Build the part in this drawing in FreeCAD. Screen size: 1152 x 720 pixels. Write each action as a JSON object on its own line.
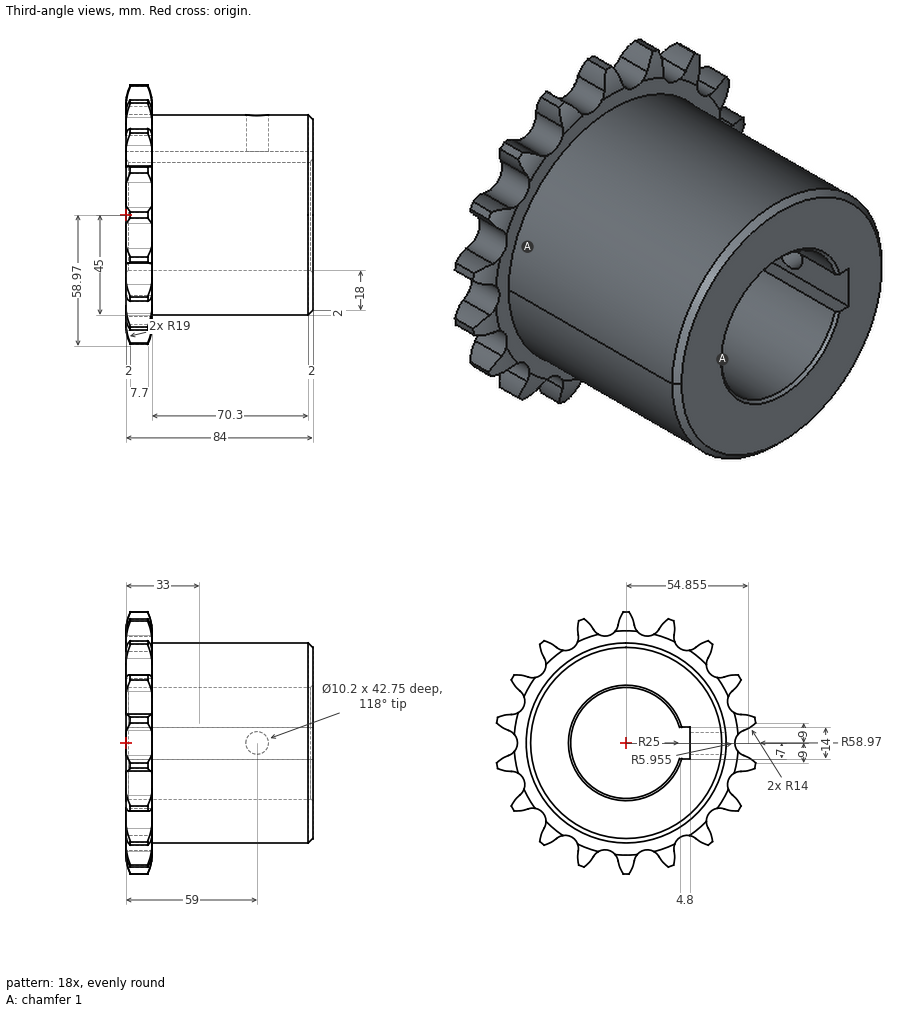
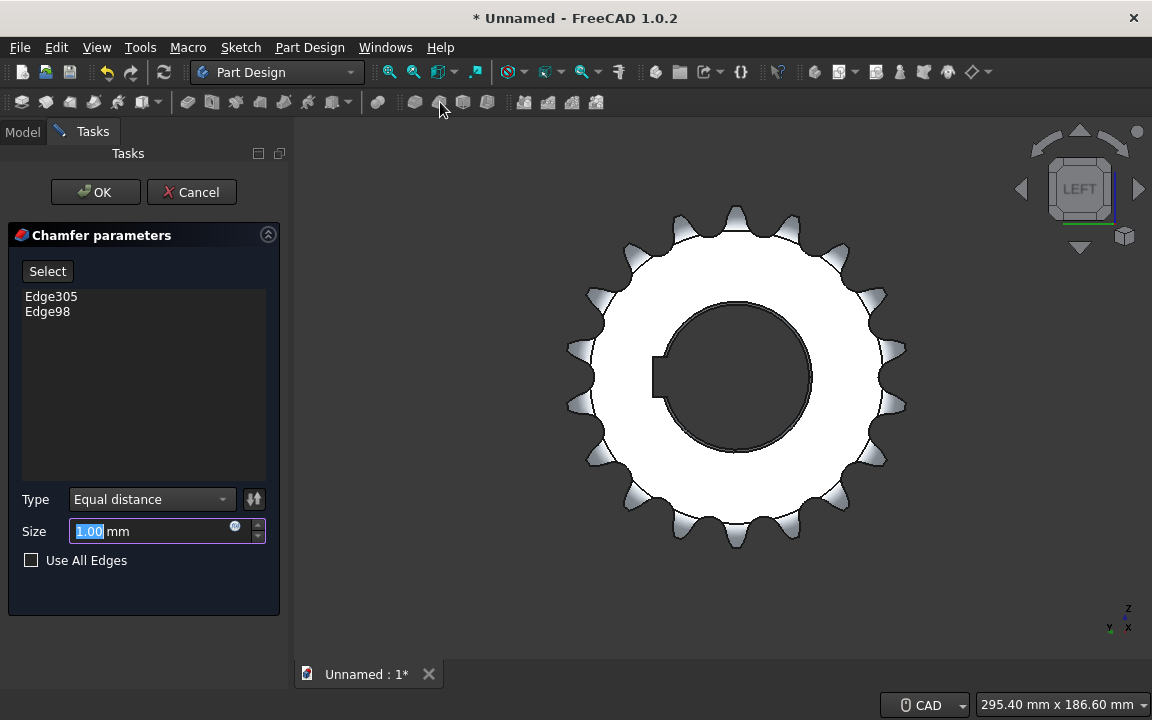
{"action": "type", "text": "1"}
{"action": "key", "text": "Tab"}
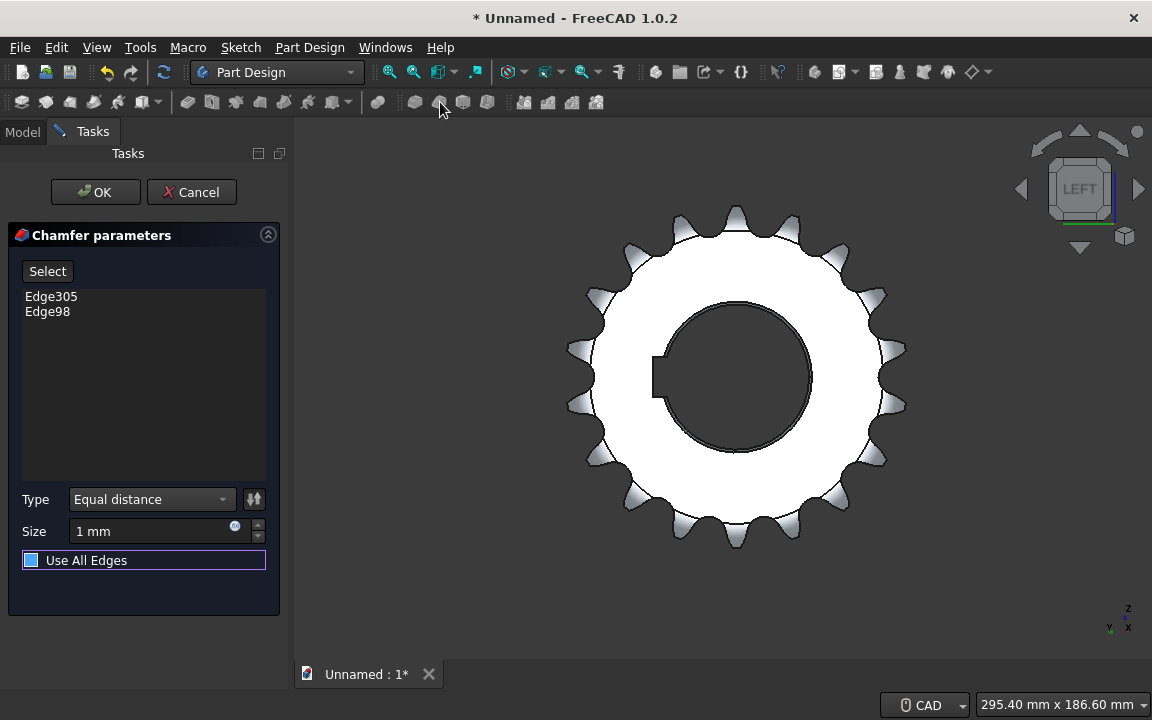
{"action": "left_click", "coordinate": [96, 192]}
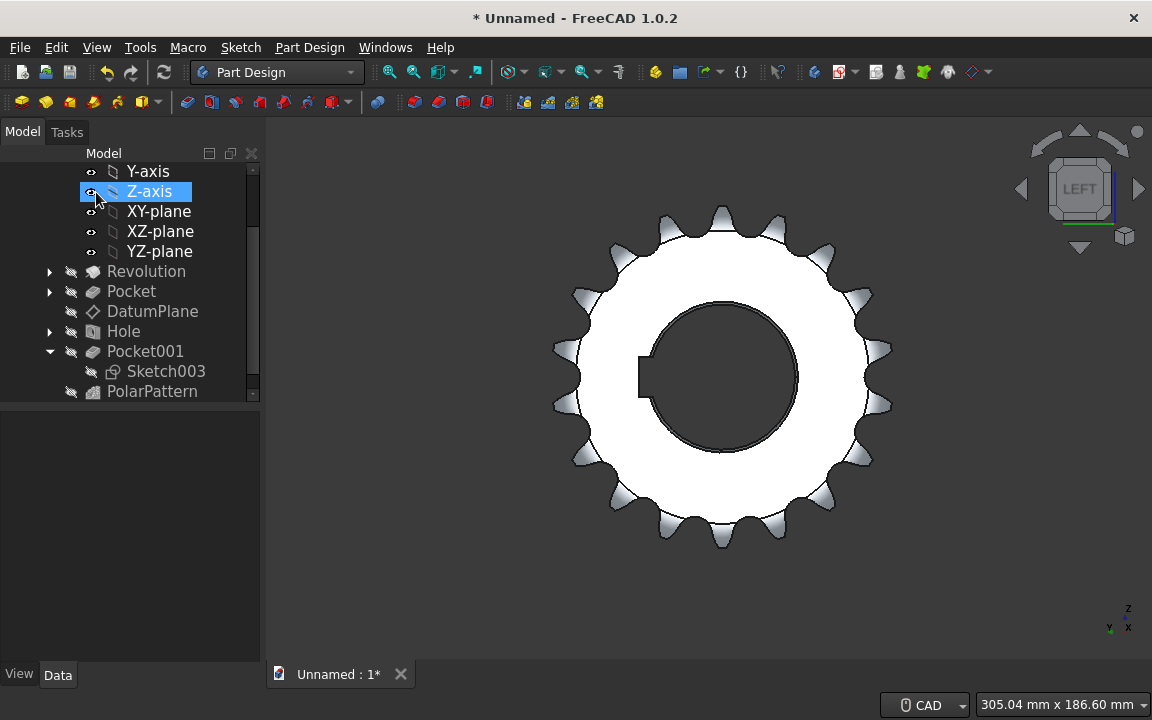
{"action": "key", "text": "0"}